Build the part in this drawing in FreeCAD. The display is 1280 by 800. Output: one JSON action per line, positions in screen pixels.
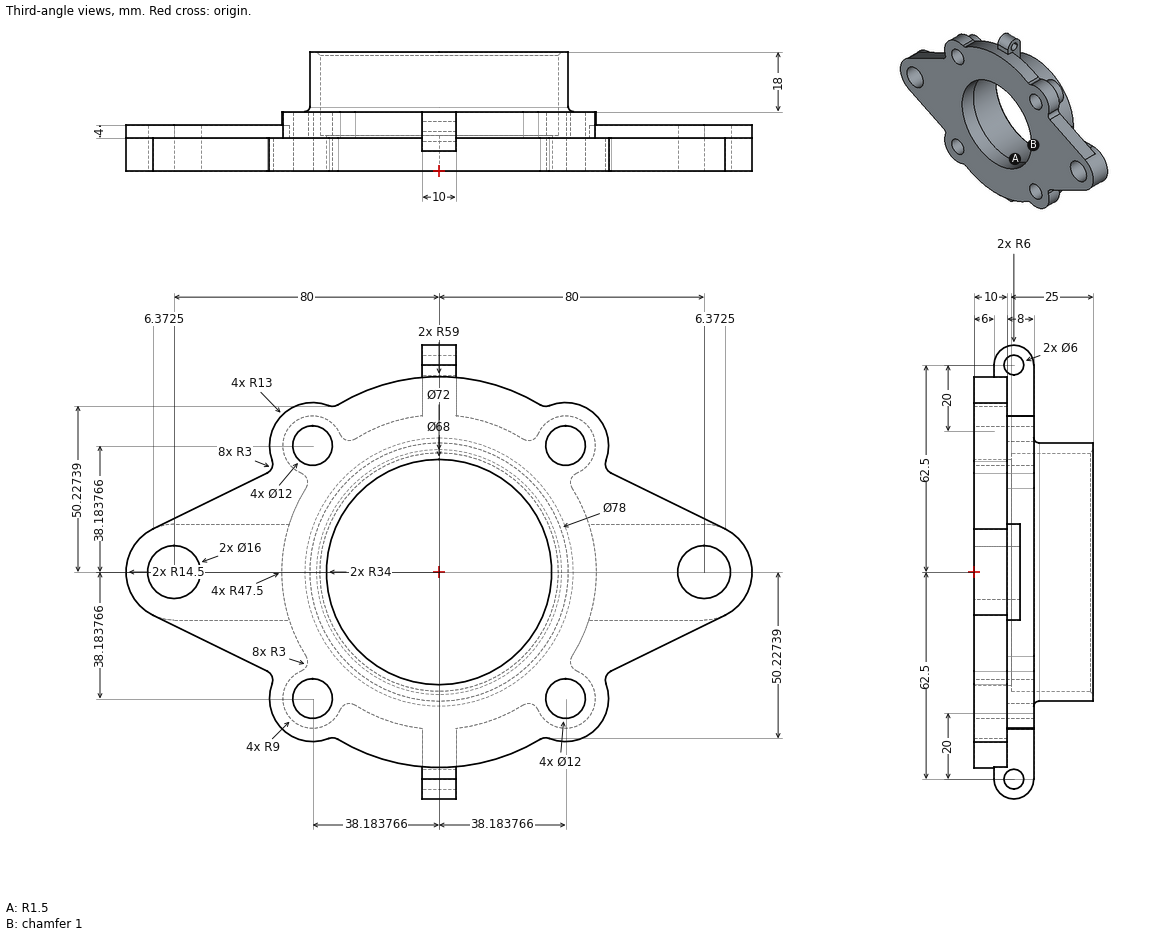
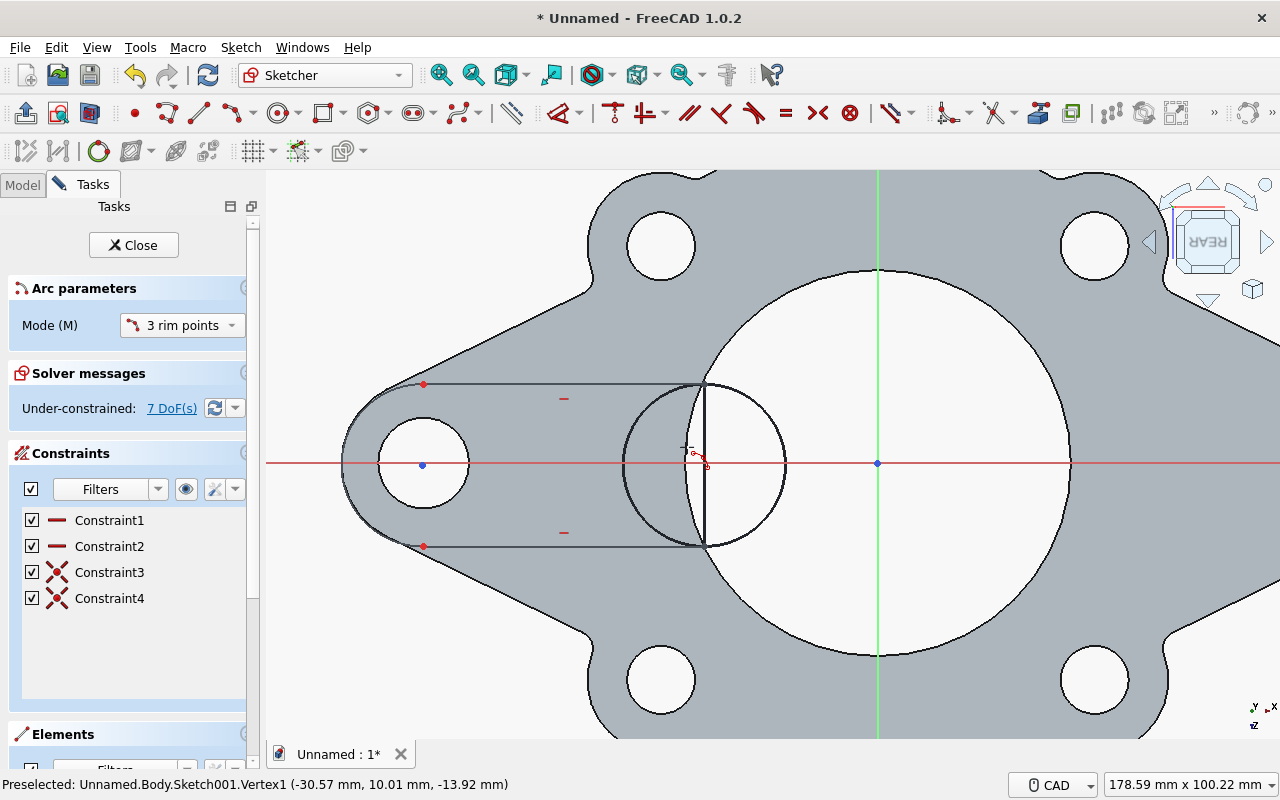
{"action": "left_click", "coordinate": [686, 446]}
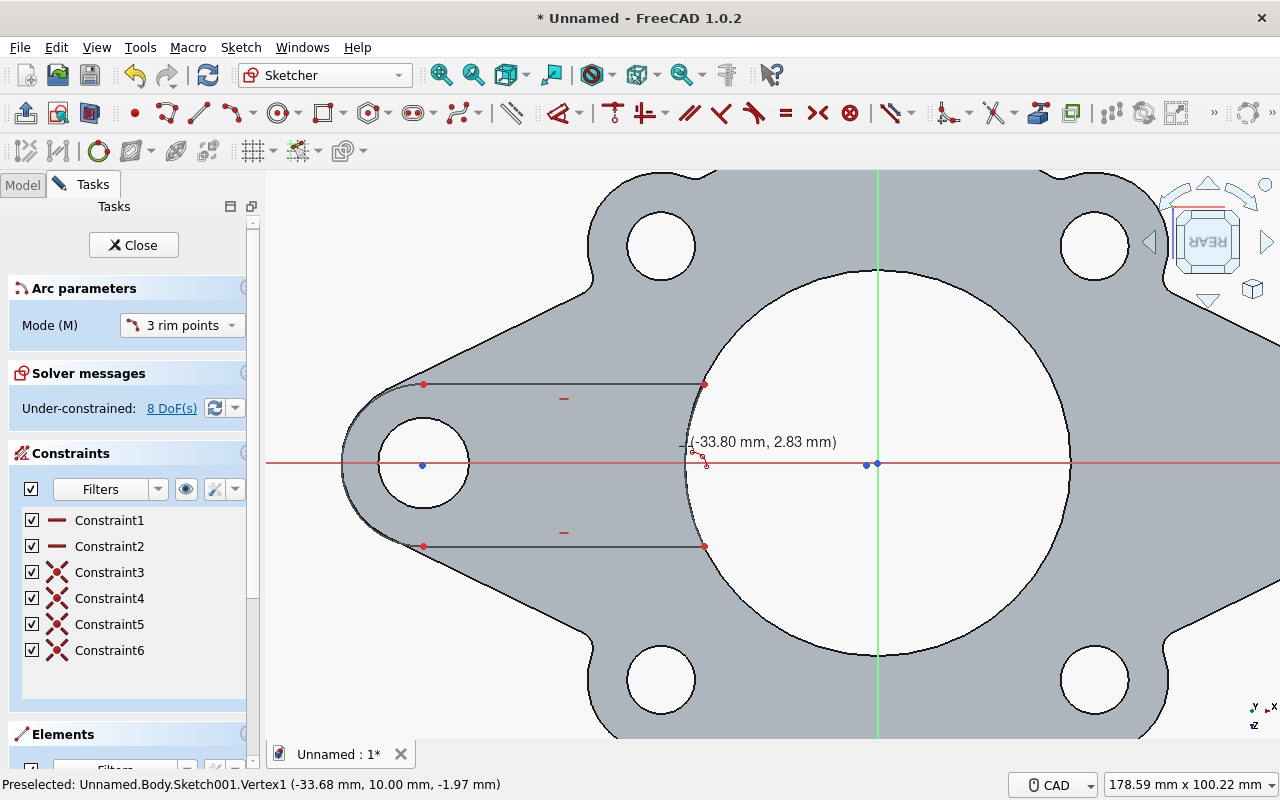
{"action": "left_click", "coordinate": [200, 114]}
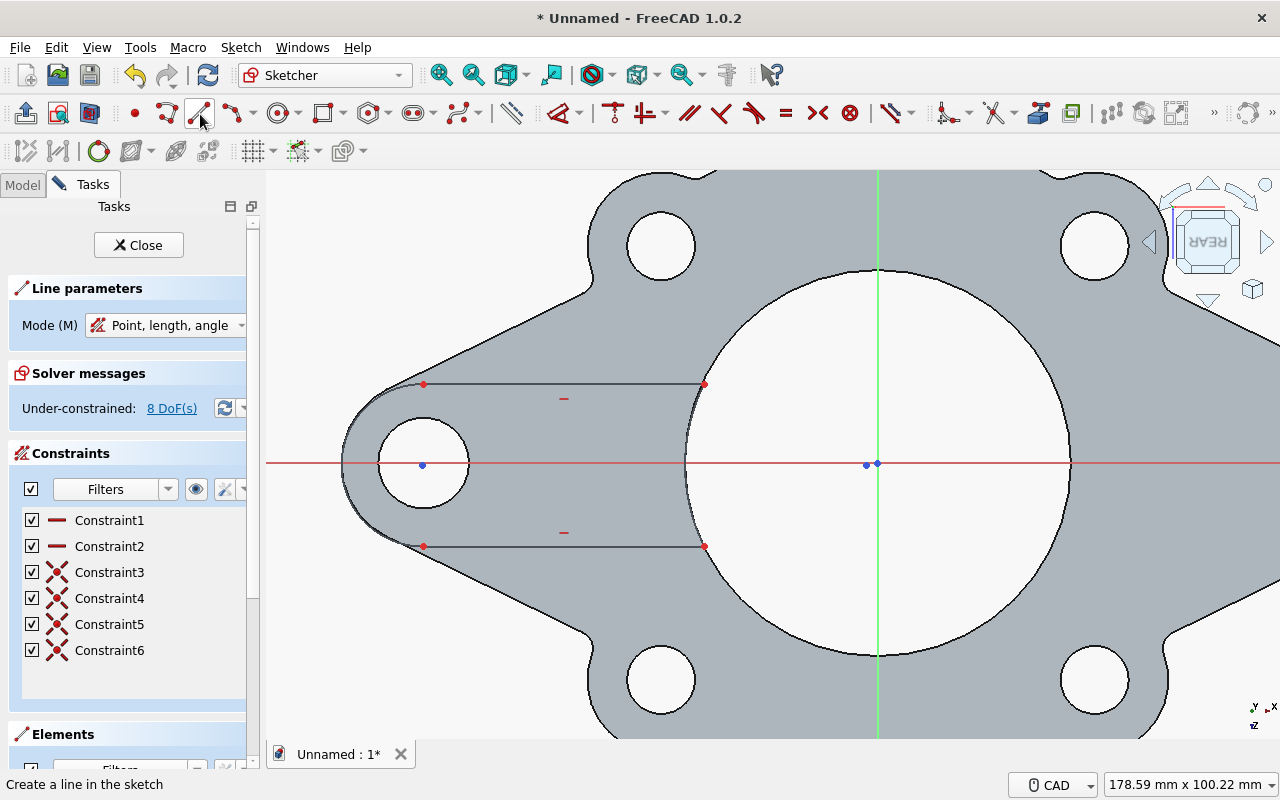
{"action": "left_click", "coordinate": [1052, 545]}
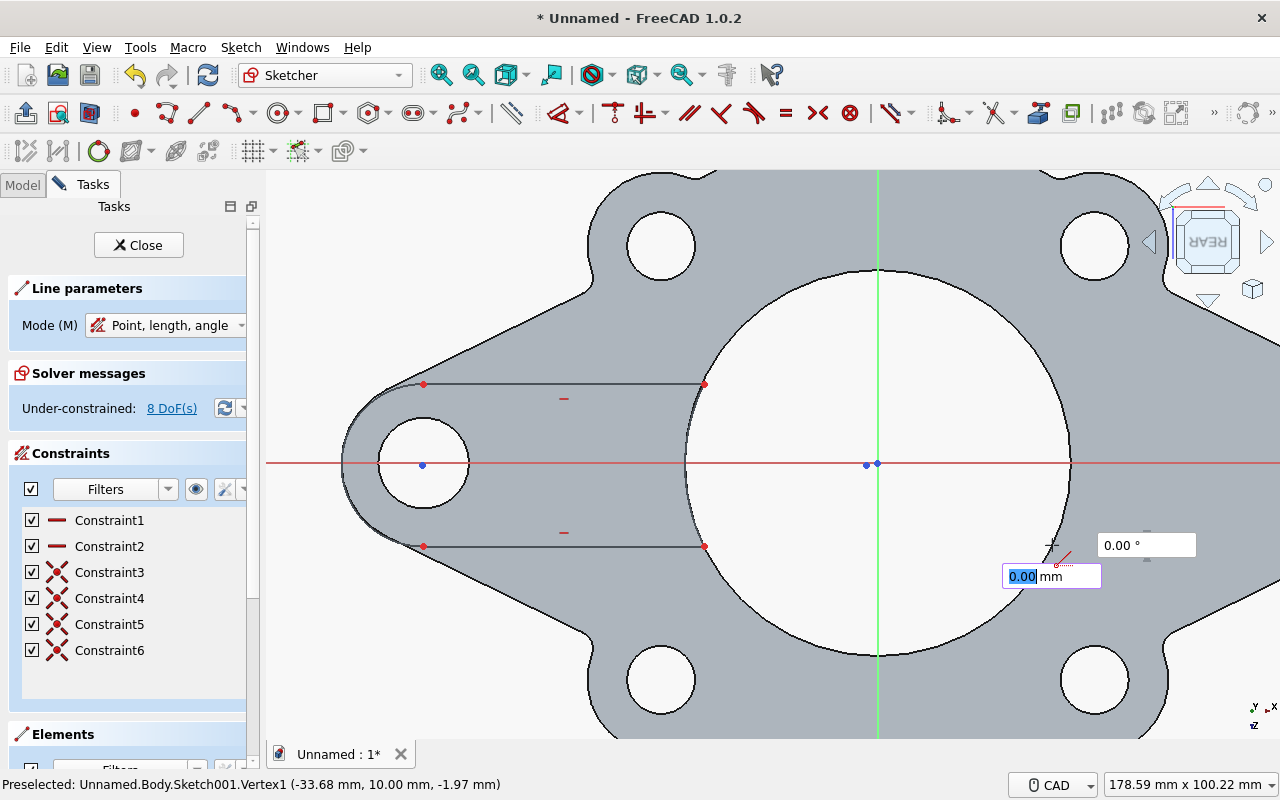
{"action": "scroll", "coordinate": [494, 444], "scroll_direction": "down", "scroll_amount": 3}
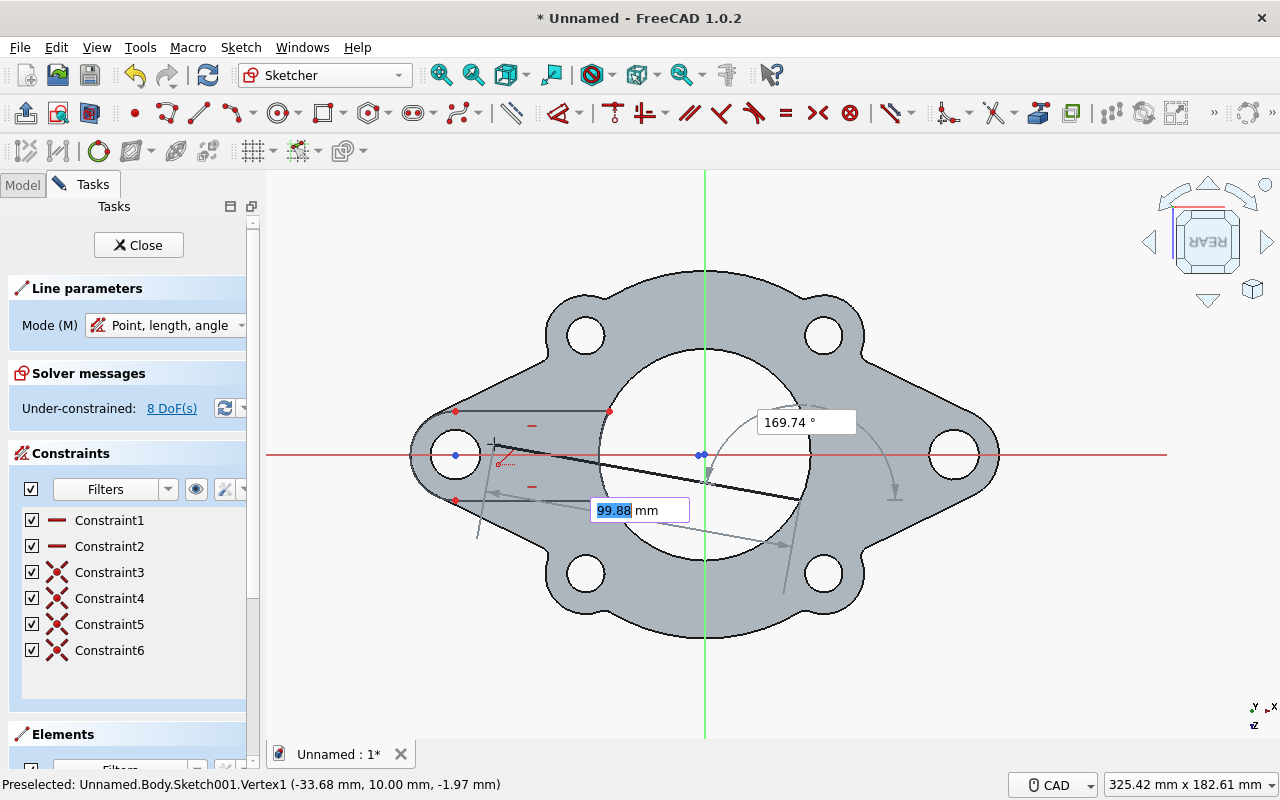
{"action": "left_click", "coordinate": [954, 500]}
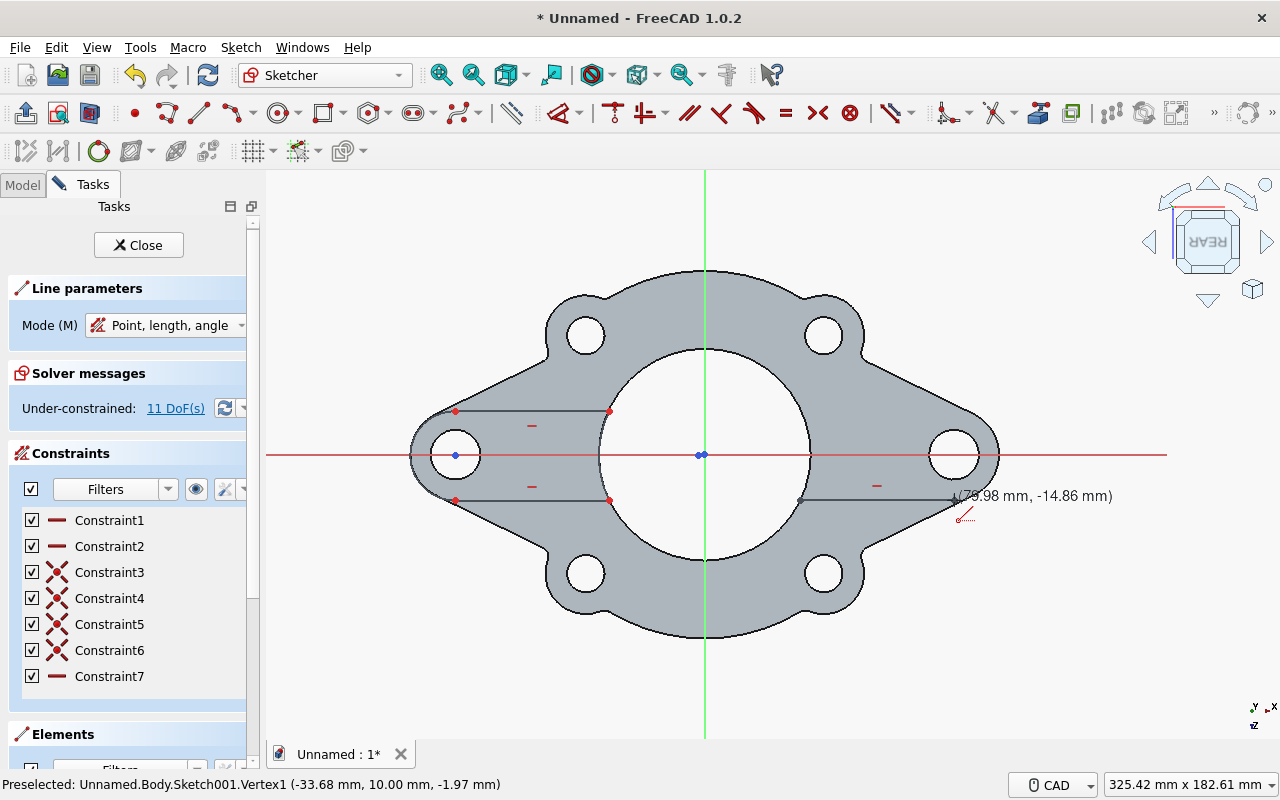
{"action": "left_click", "coordinate": [954, 410]}
{"action": "left_click", "coordinate": [801, 410]}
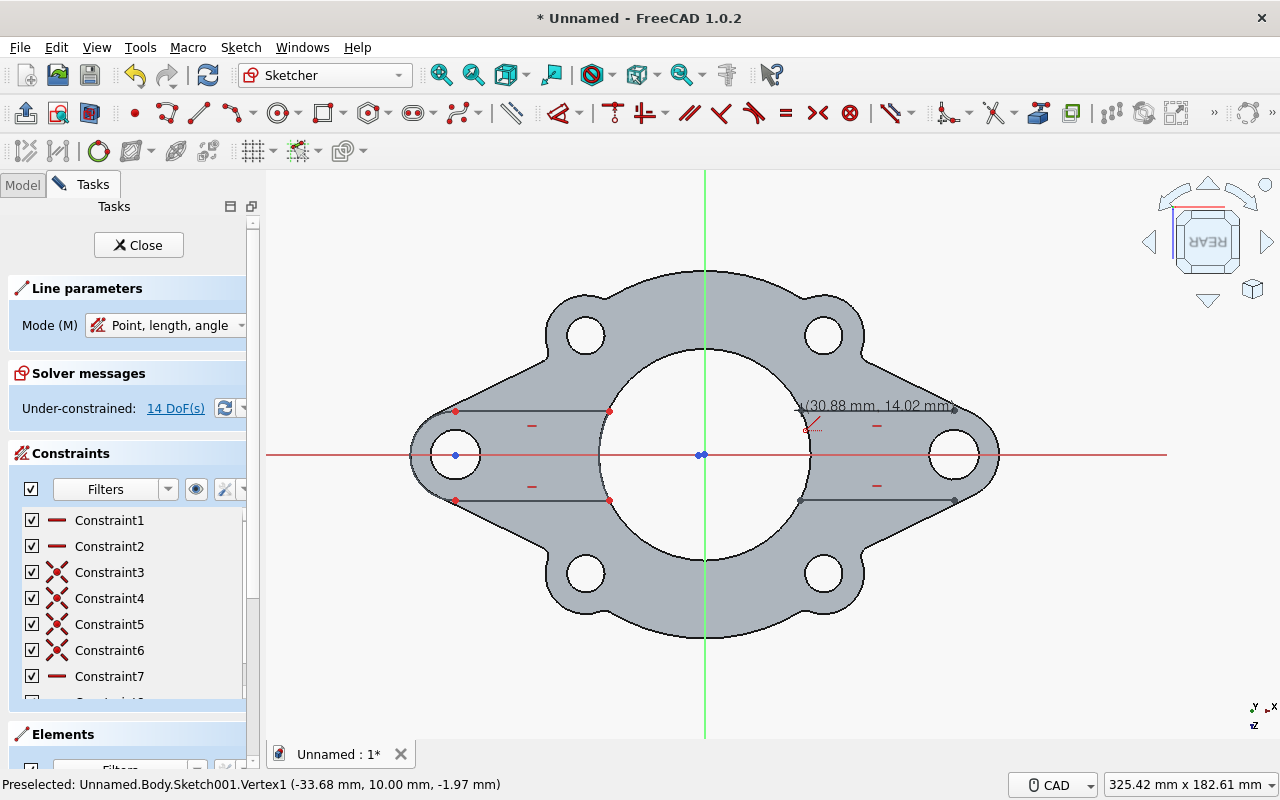
{"action": "left_click", "coordinate": [232, 114]}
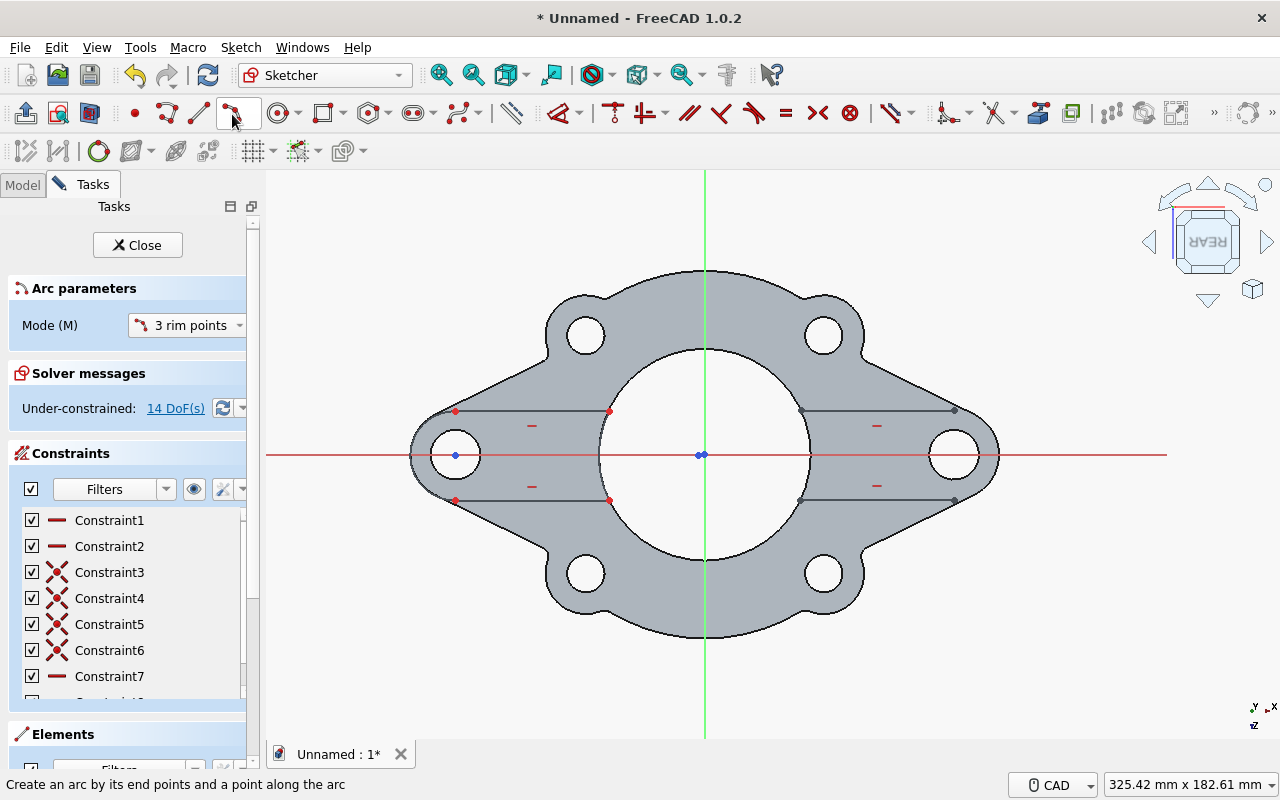
{"action": "left_click", "coordinate": [954, 500]}
{"action": "left_click", "coordinate": [954, 411]}
{"action": "left_click", "coordinate": [991, 481]}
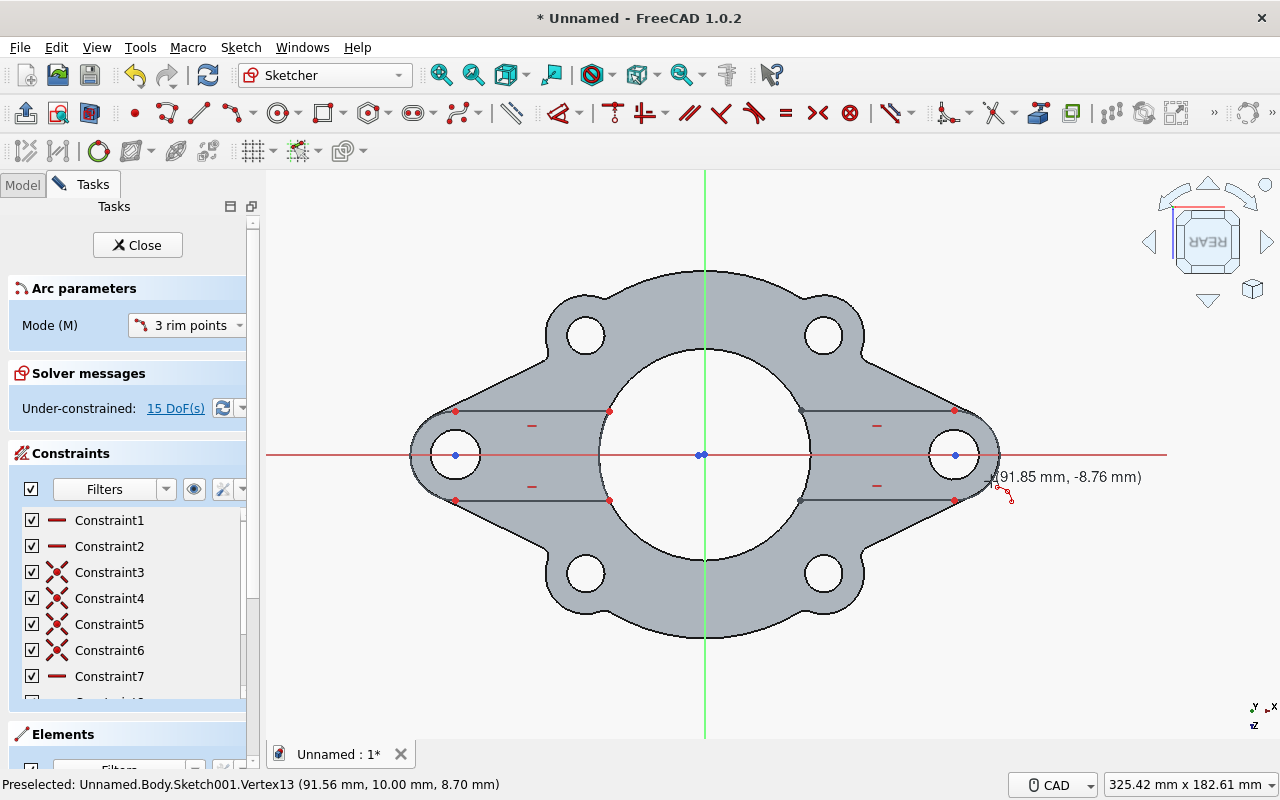
{"action": "left_click", "coordinate": [801, 411]}
{"action": "left_click", "coordinate": [800, 500]}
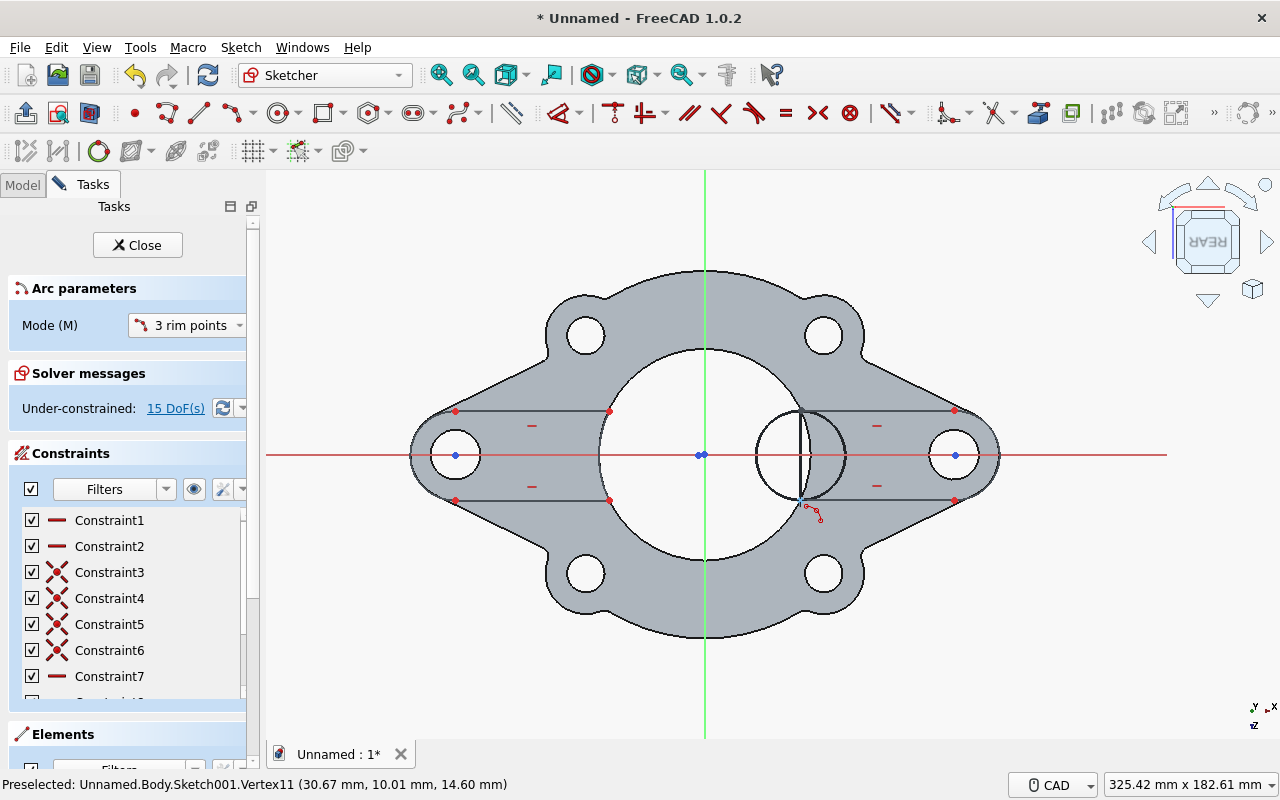
{"action": "scroll", "coordinate": [810, 445], "scroll_direction": "up", "scroll_amount": 3}